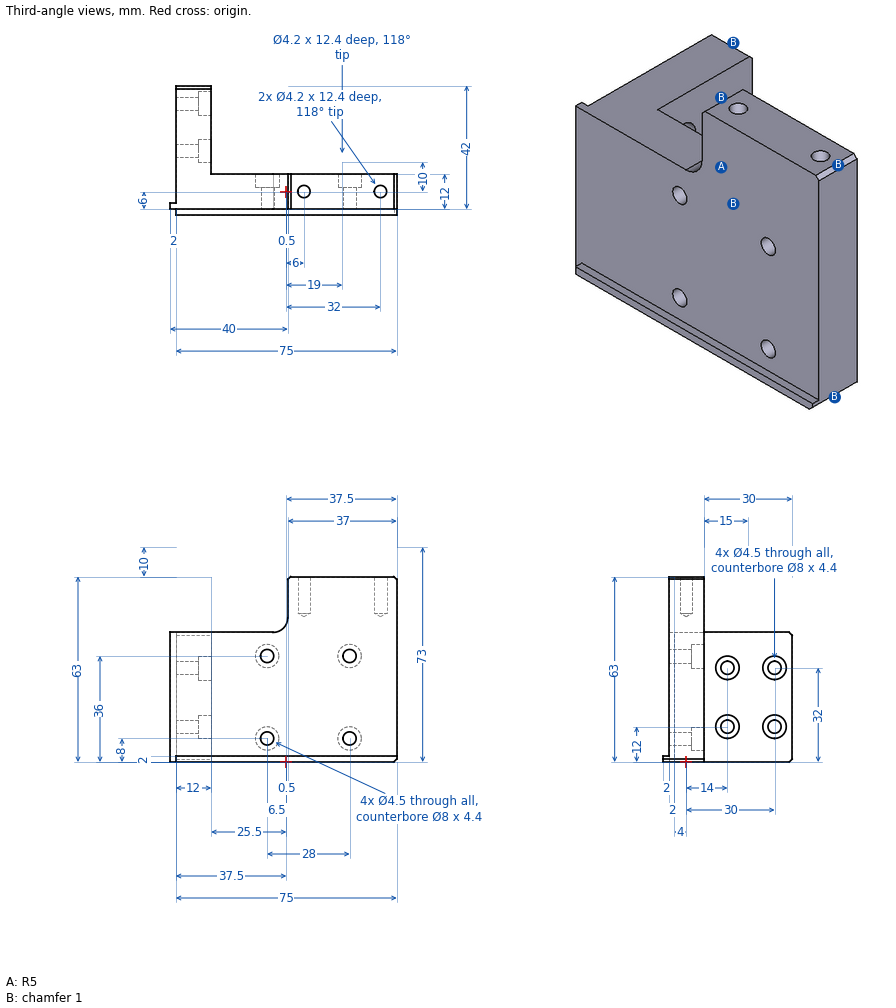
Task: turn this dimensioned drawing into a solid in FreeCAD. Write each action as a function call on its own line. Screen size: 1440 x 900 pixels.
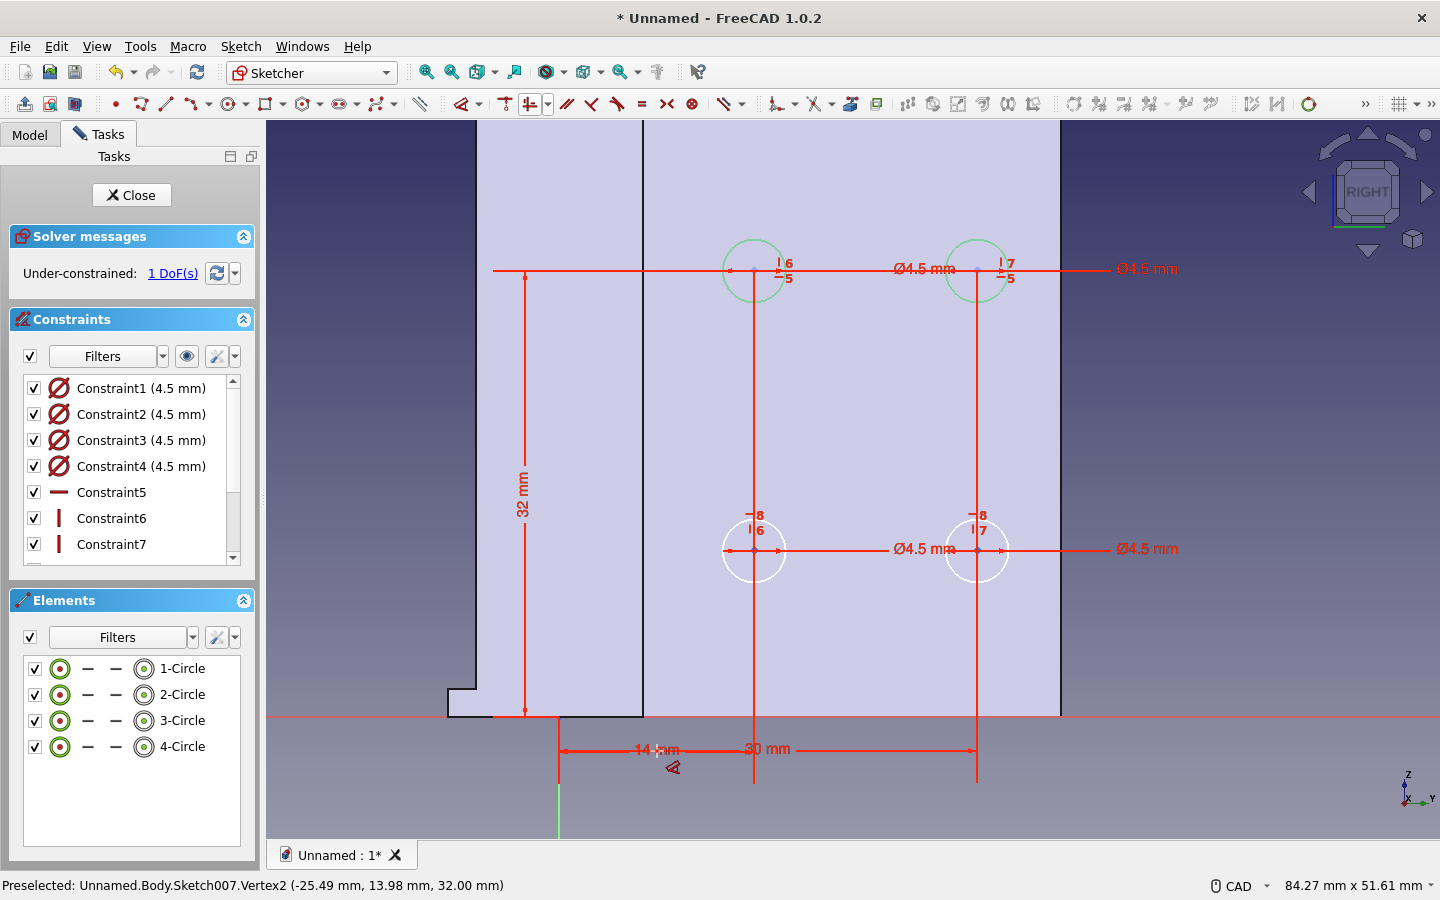
click(754, 551)
click(525, 634)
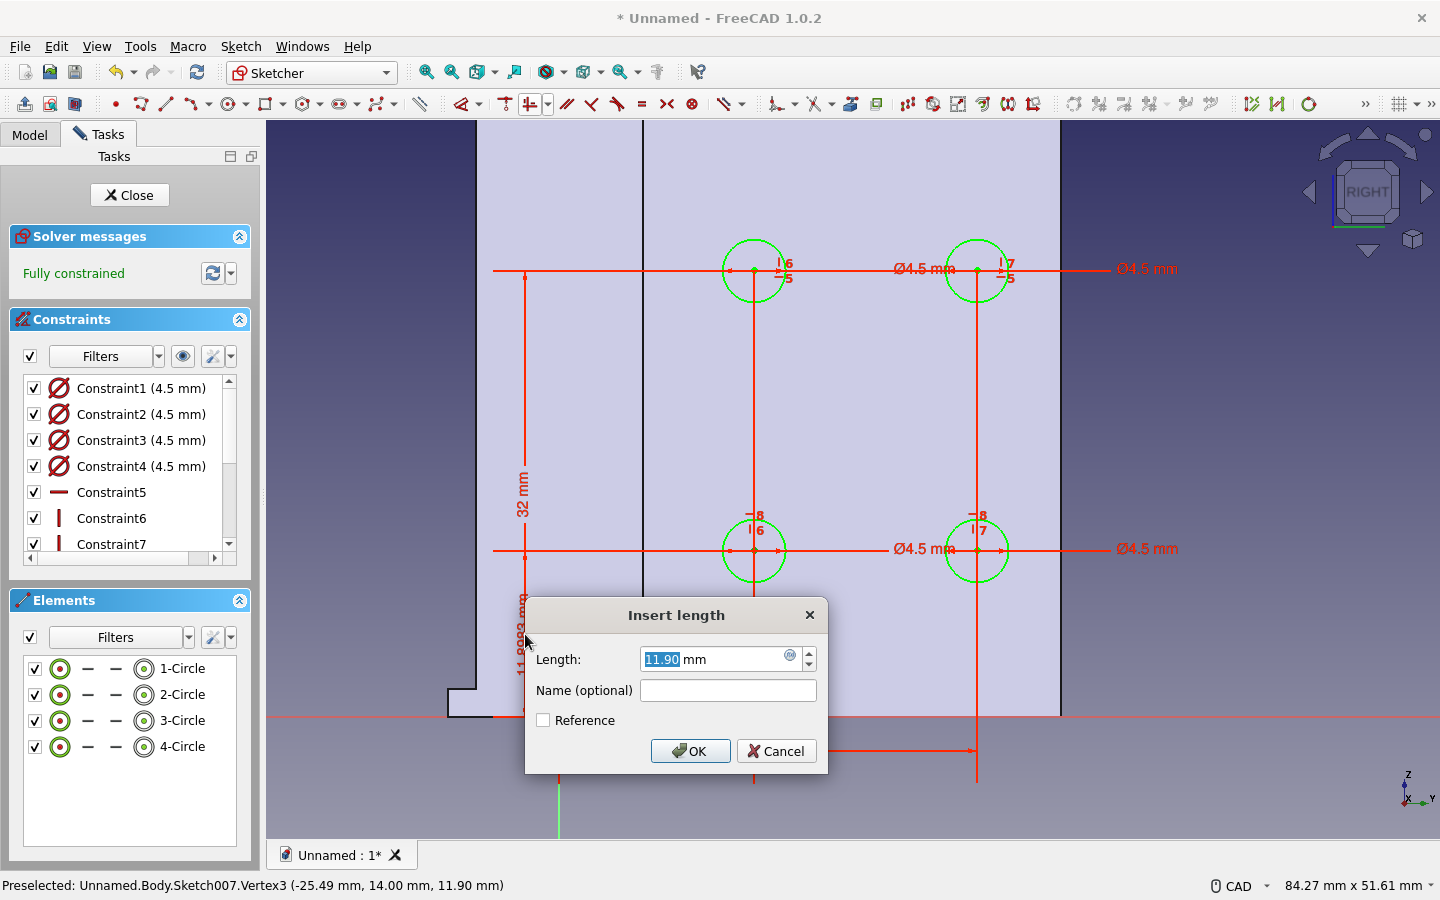
text(12)
key(Return)
key(Escape)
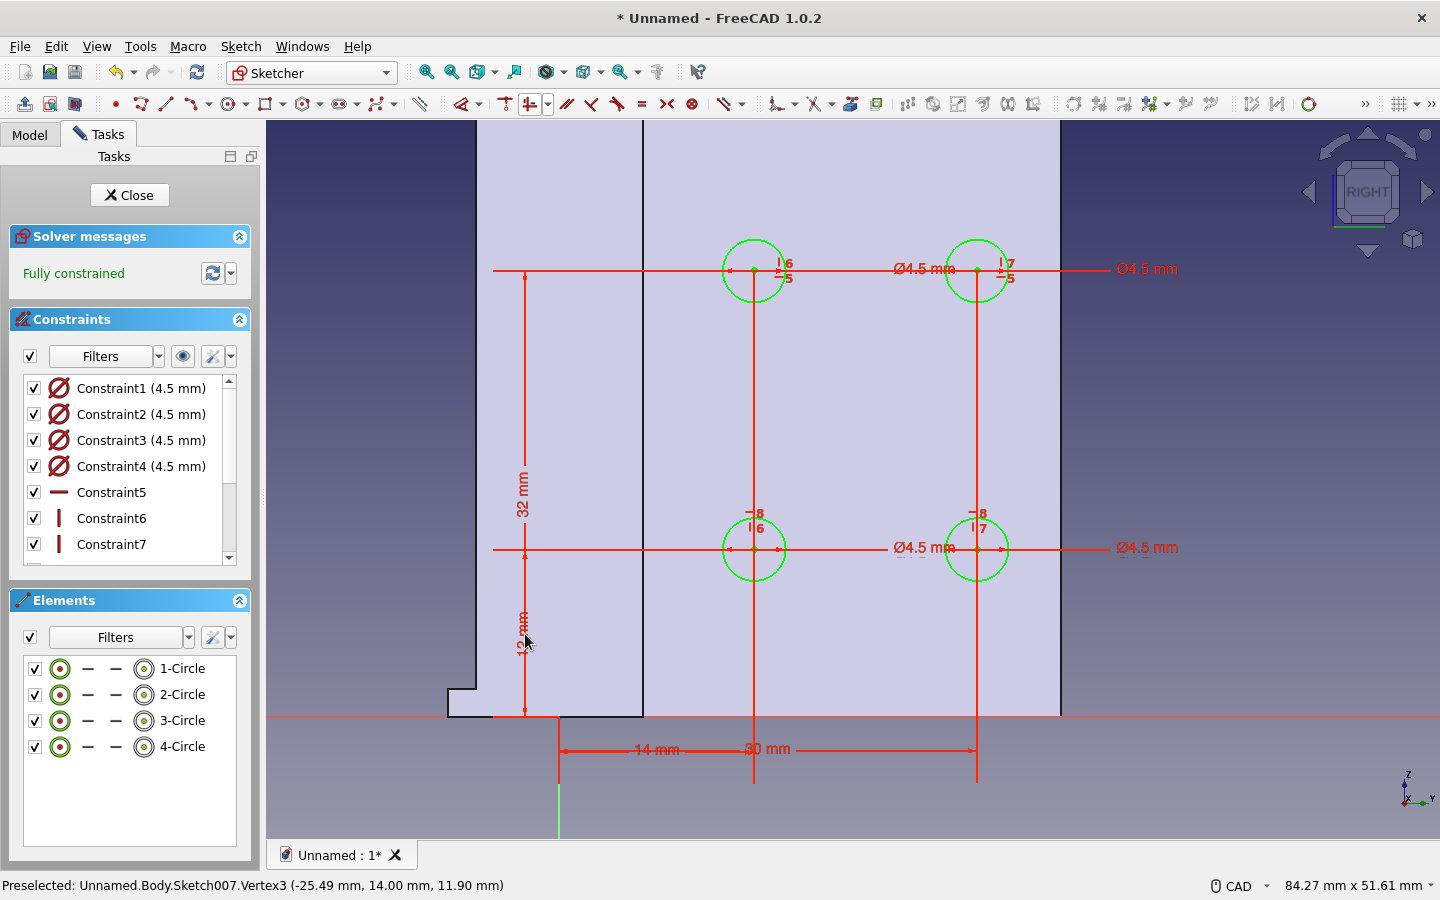
click(130, 195)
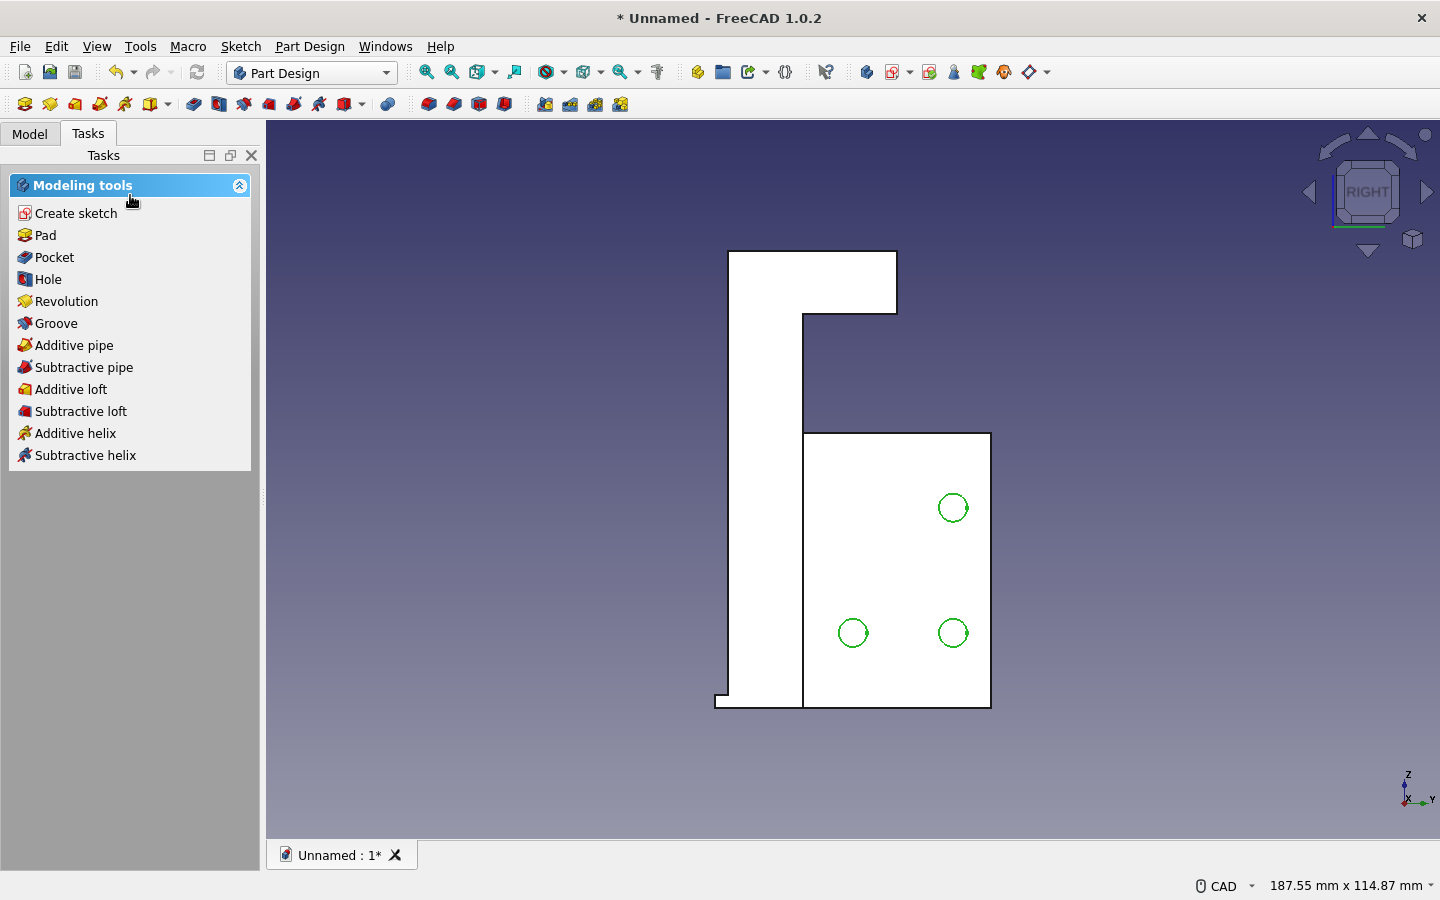
click(219, 104)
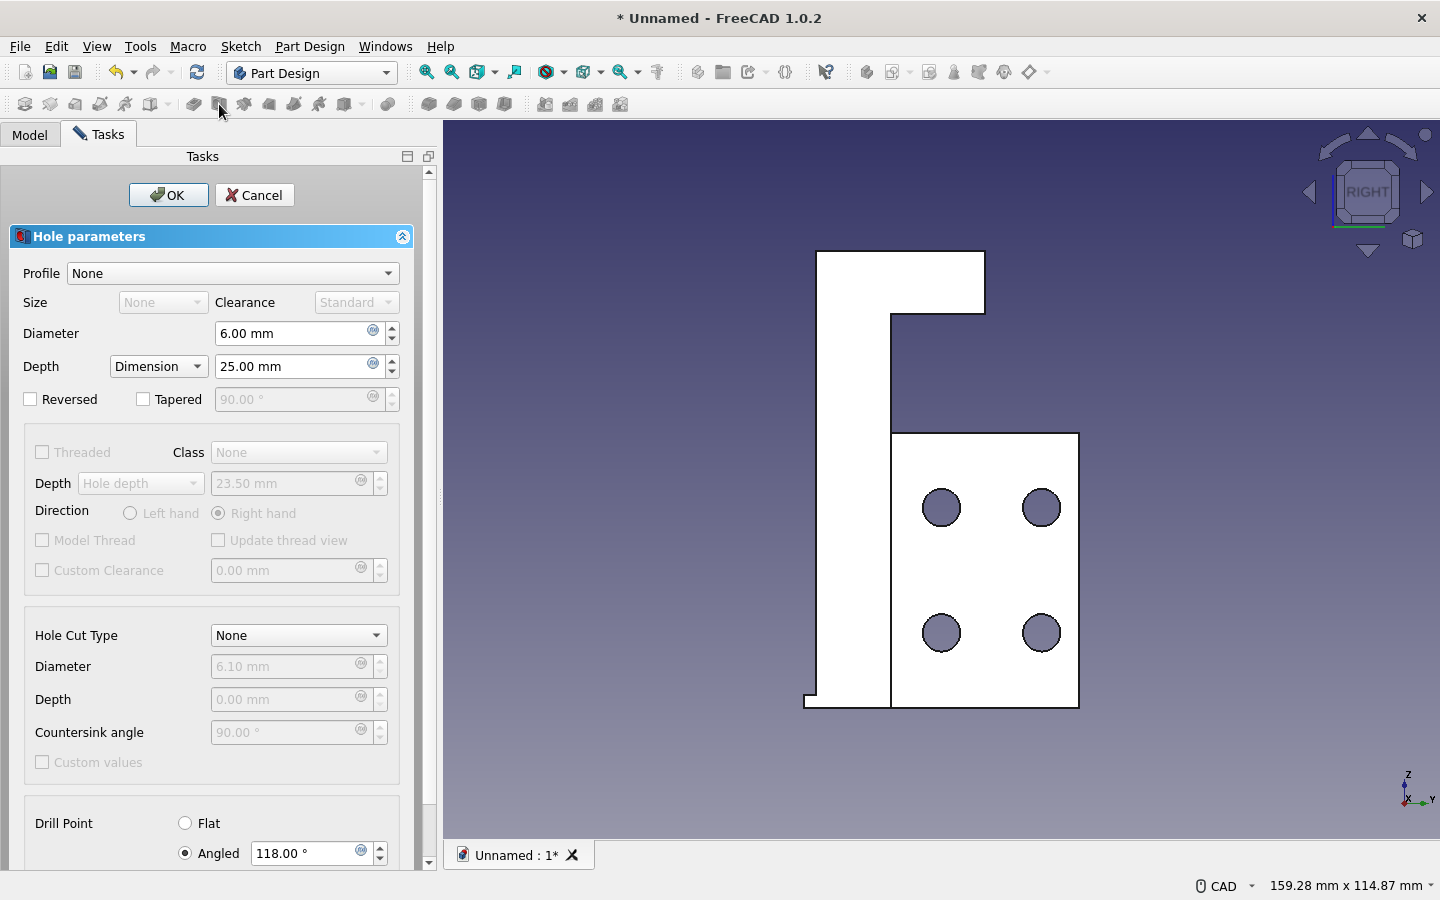
triple_click(300, 334)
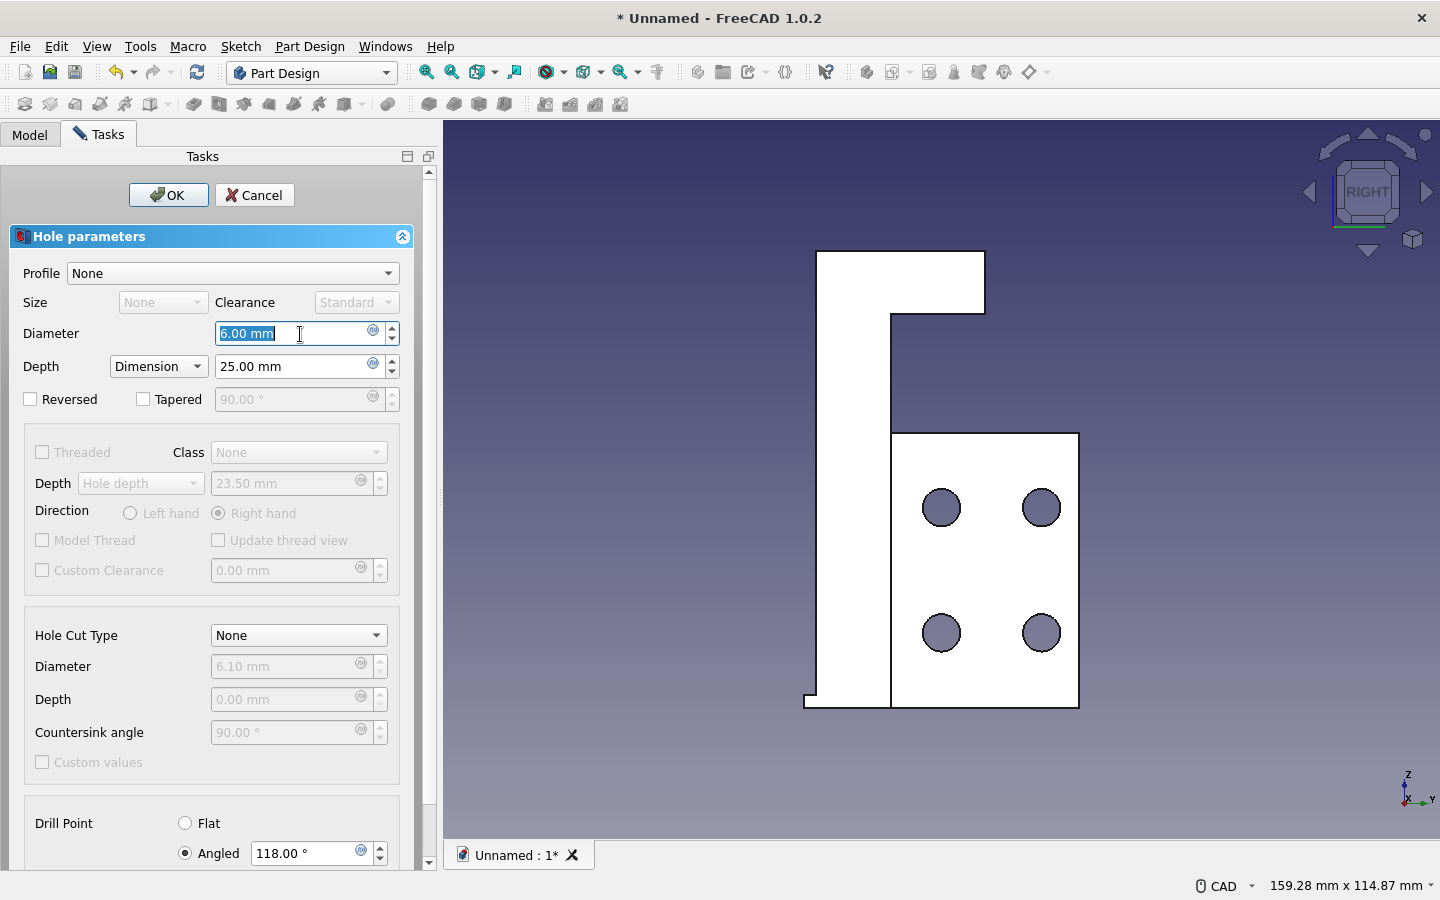
text(4.5)
key(Tab)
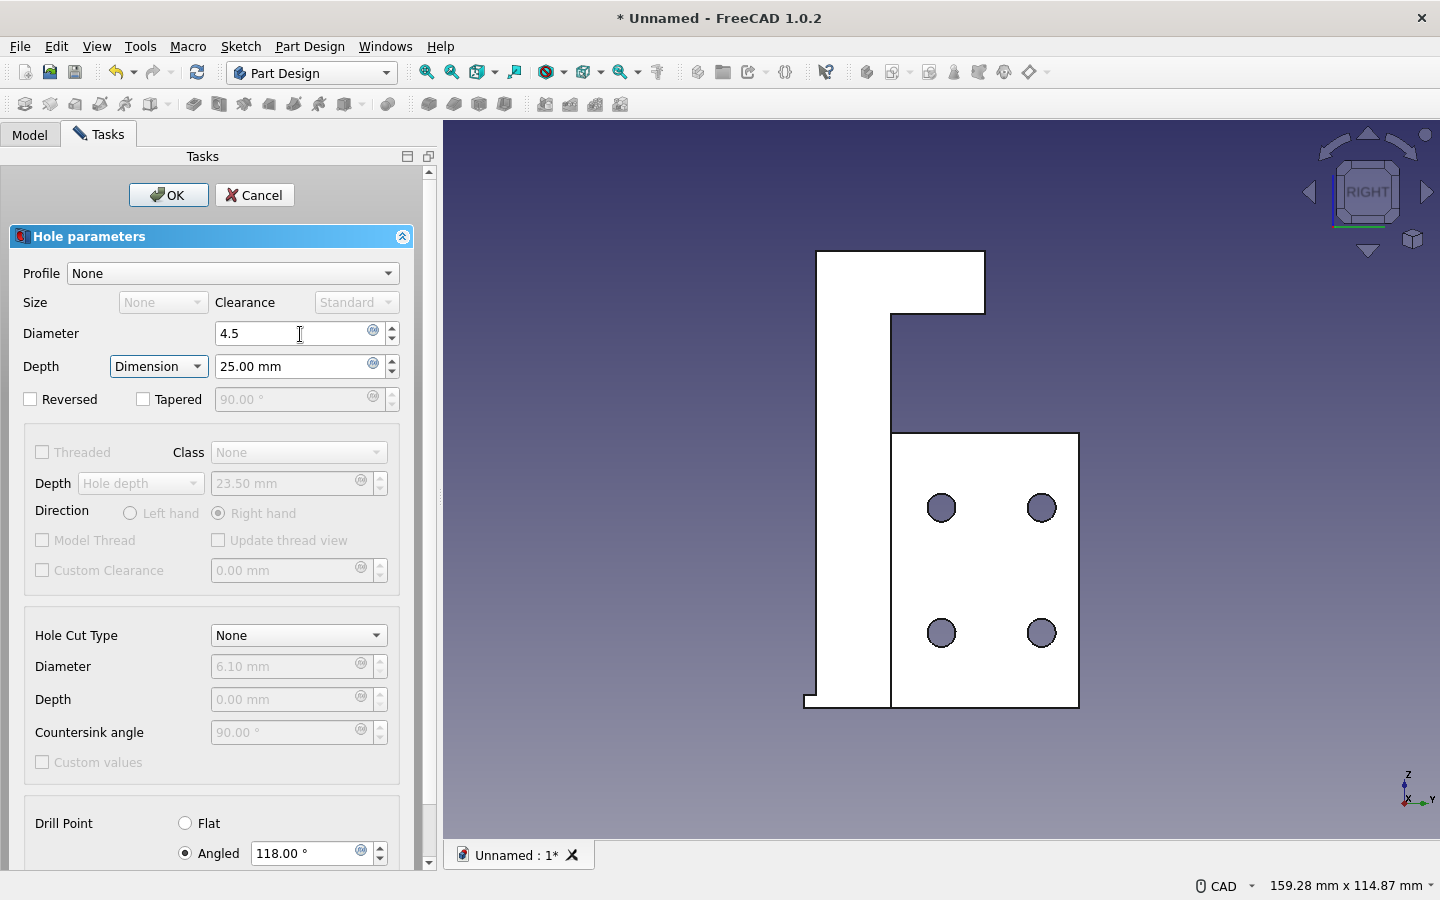
click(160, 366)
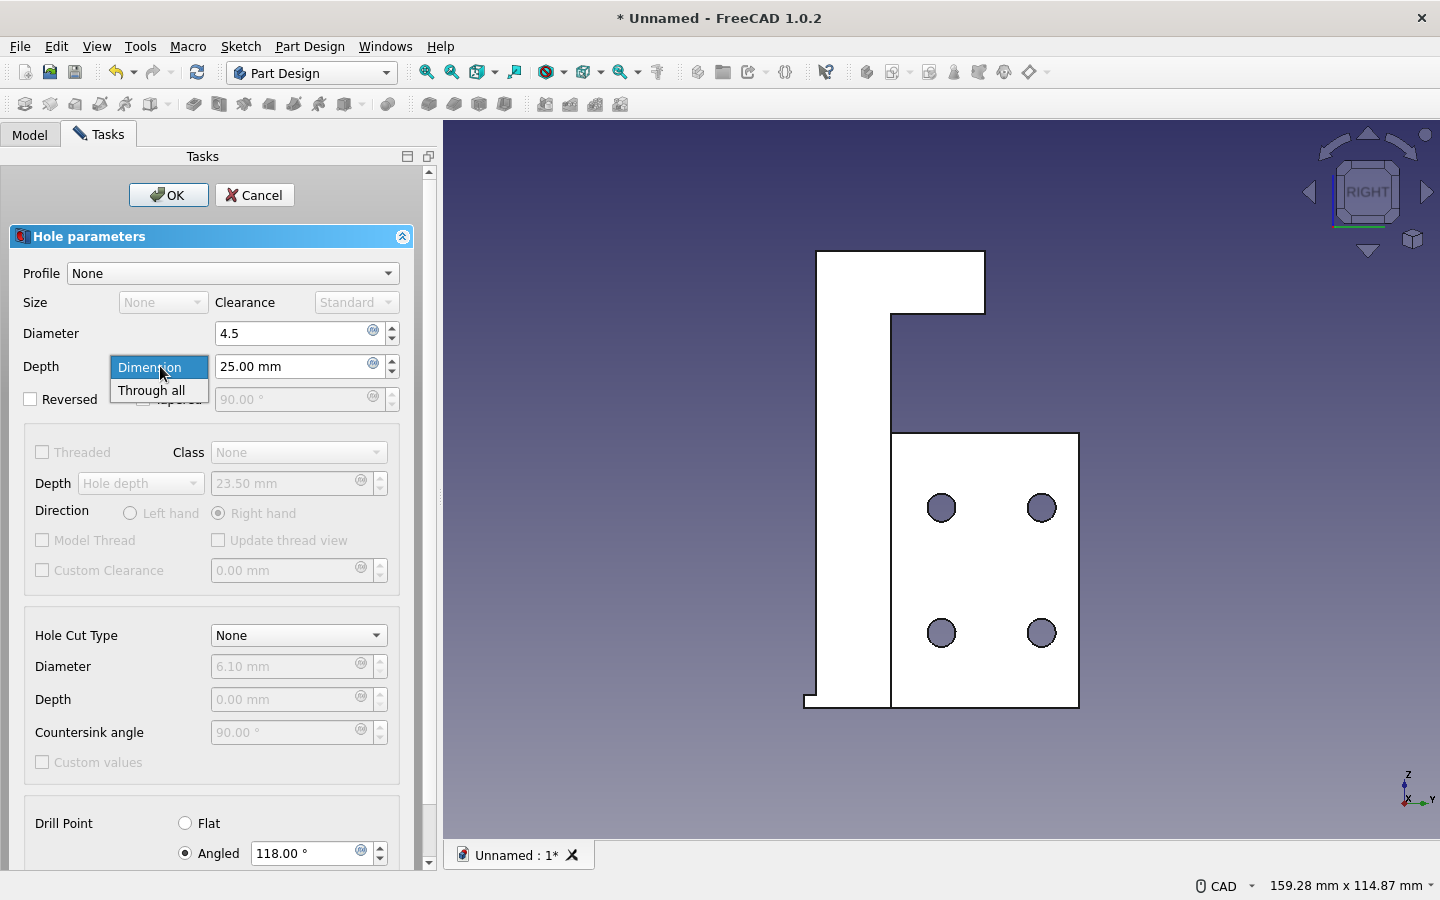
click(158, 390)